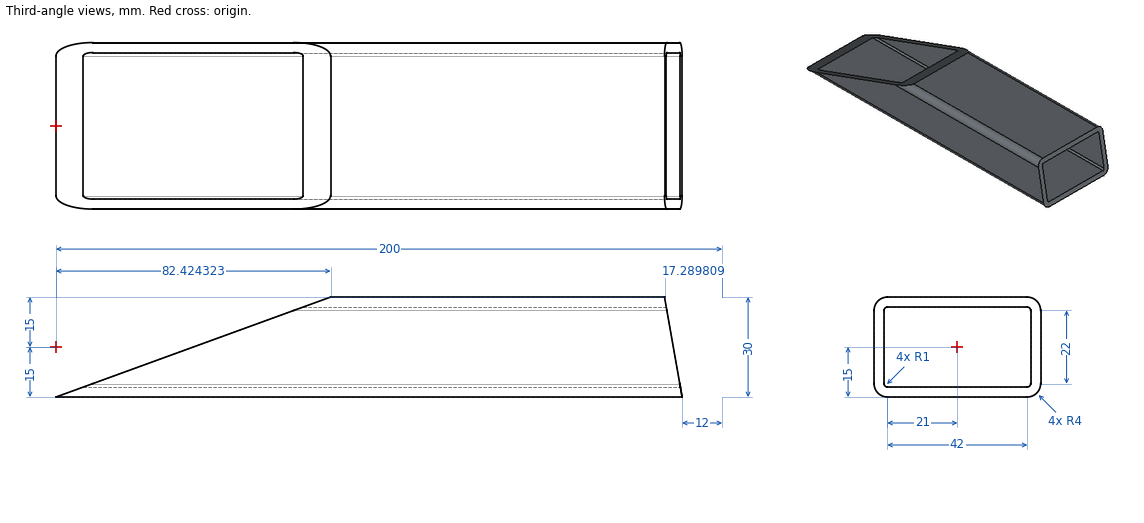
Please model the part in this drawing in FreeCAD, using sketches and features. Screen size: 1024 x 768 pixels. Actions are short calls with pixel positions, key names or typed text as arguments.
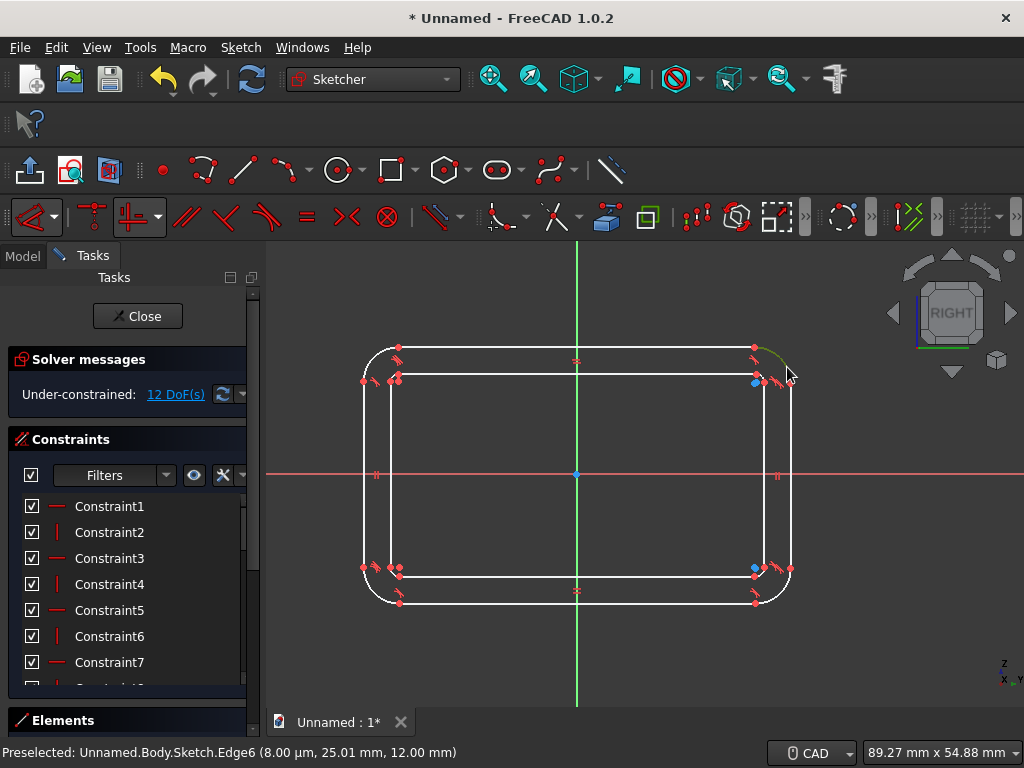
scroll(762, 377, up, 4)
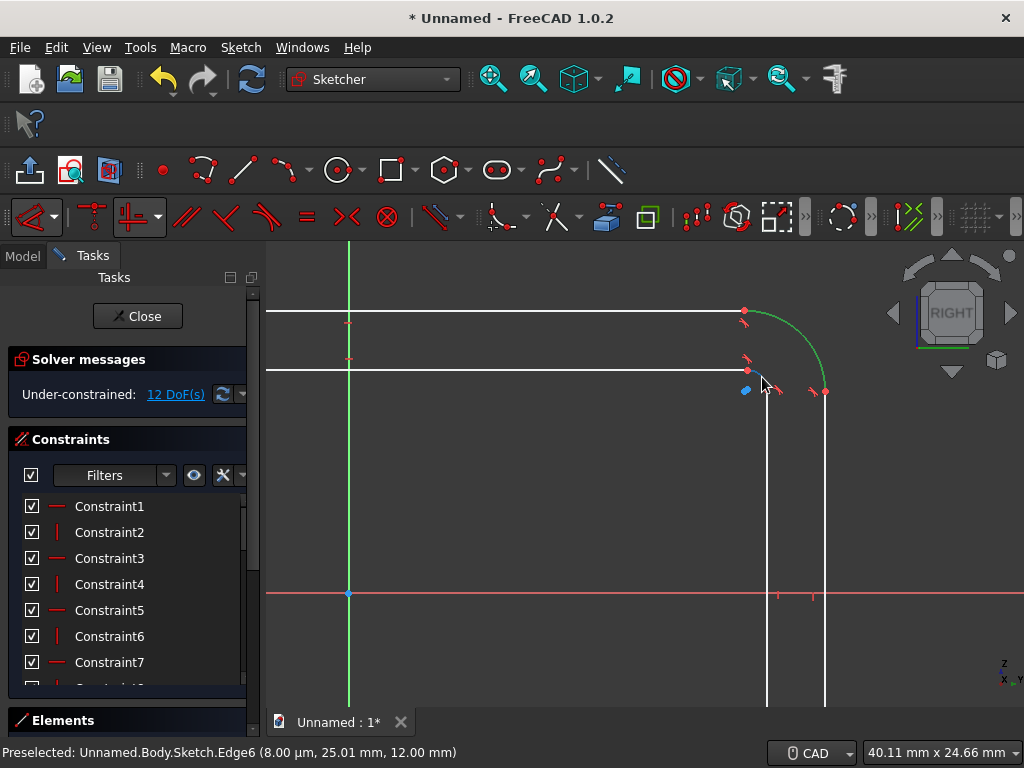
click(761, 376)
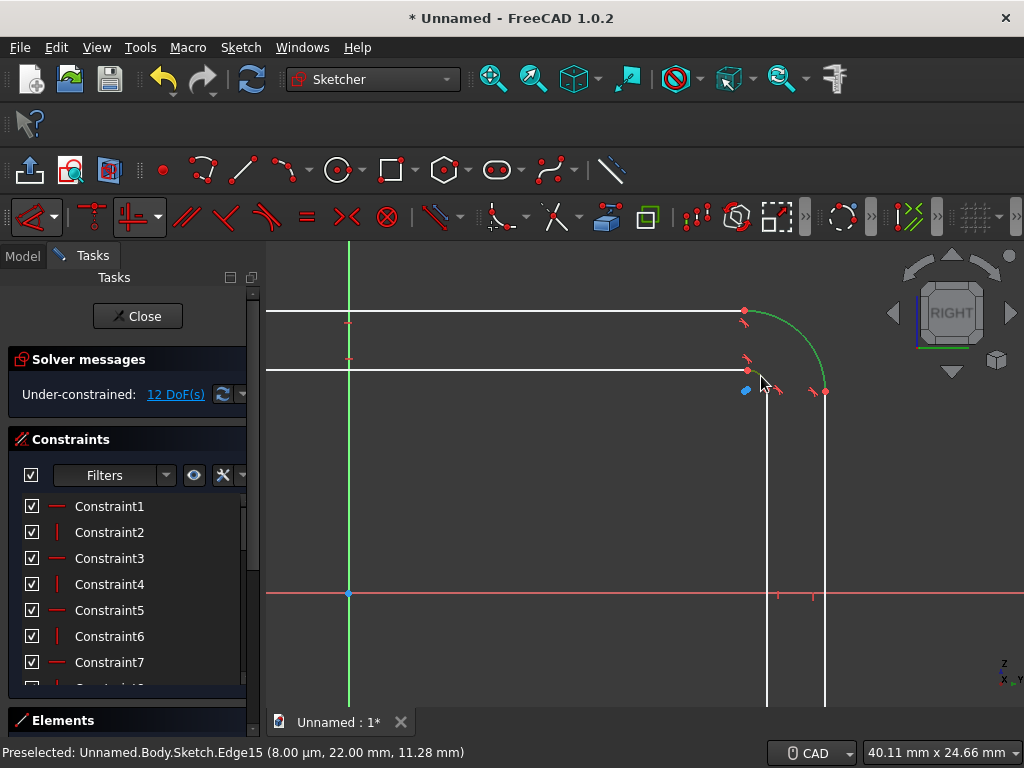
click(92, 218)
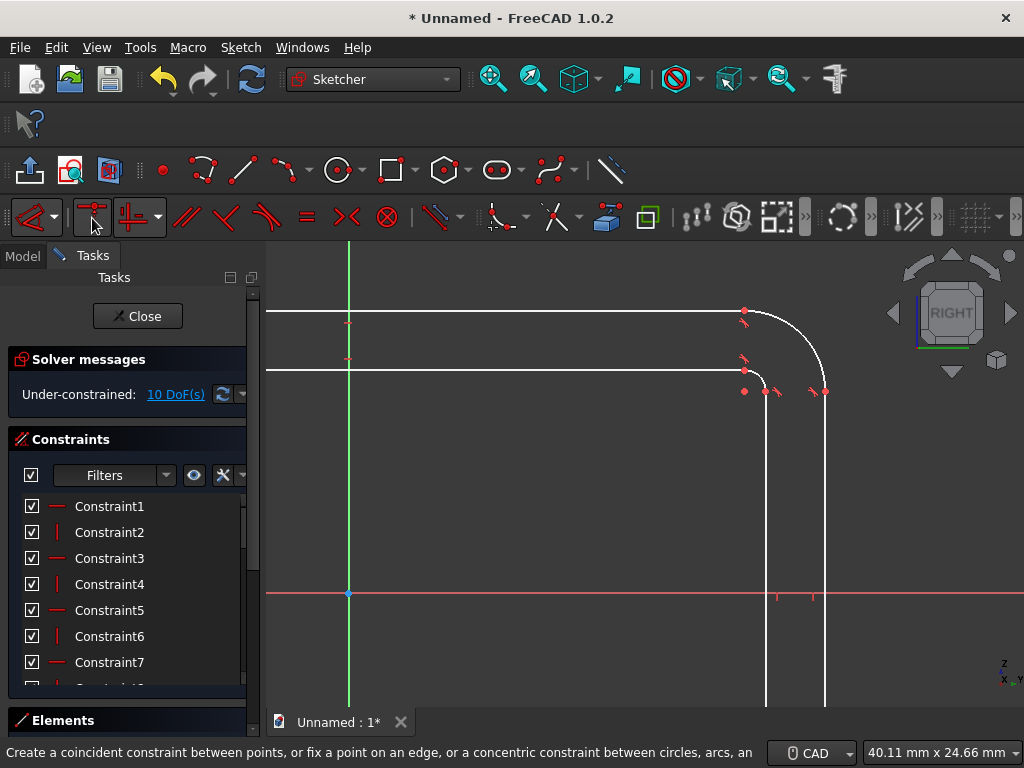
scroll(762, 377, down, 4)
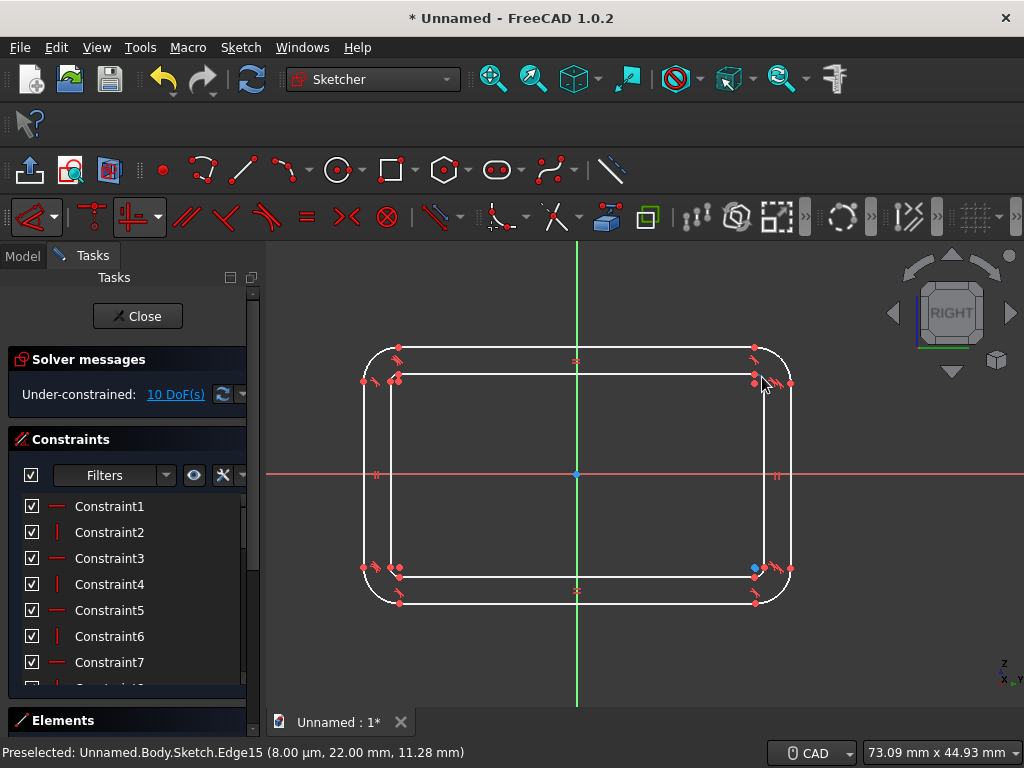
click(771, 600)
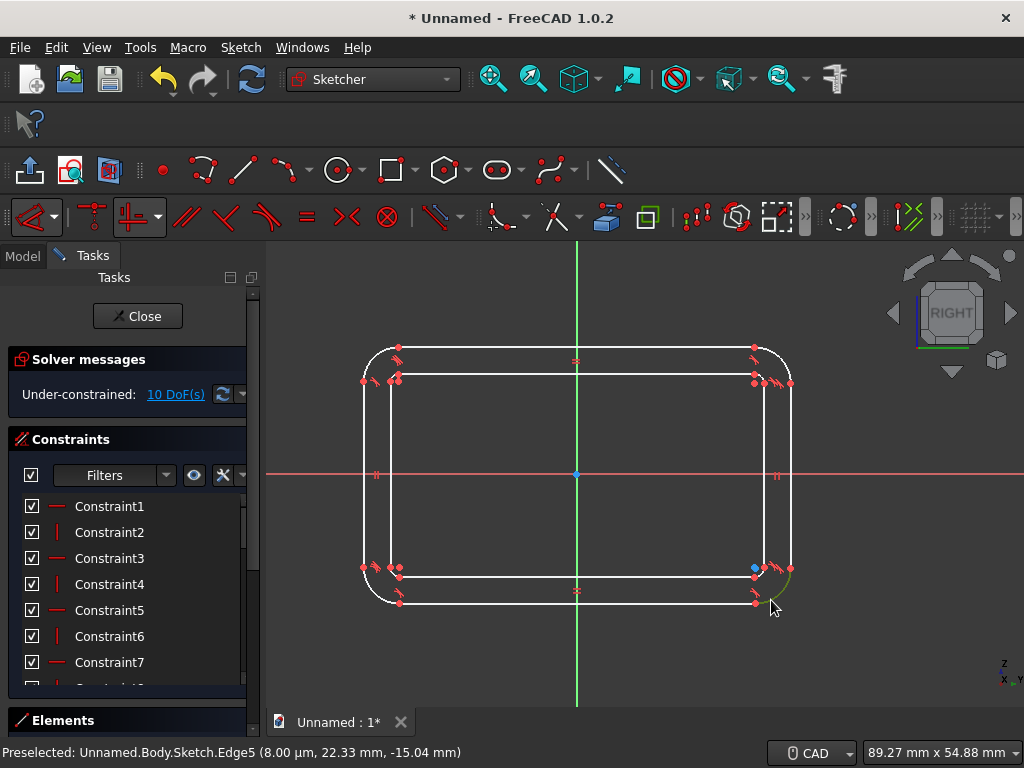
click(787, 367)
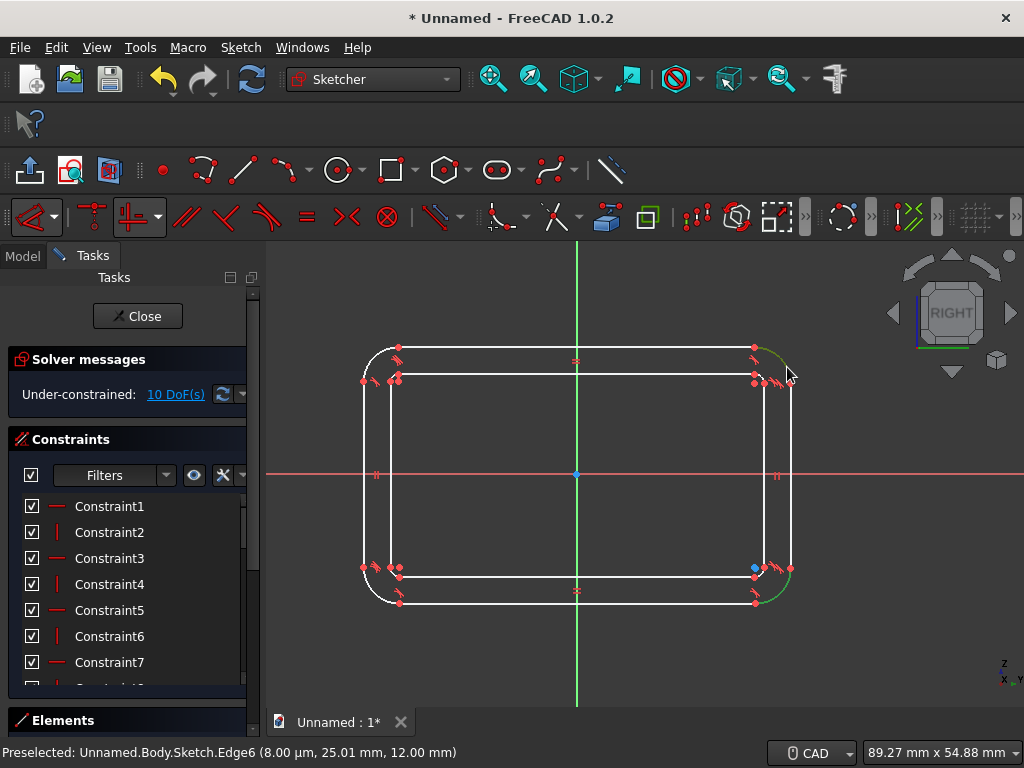
click(383, 351)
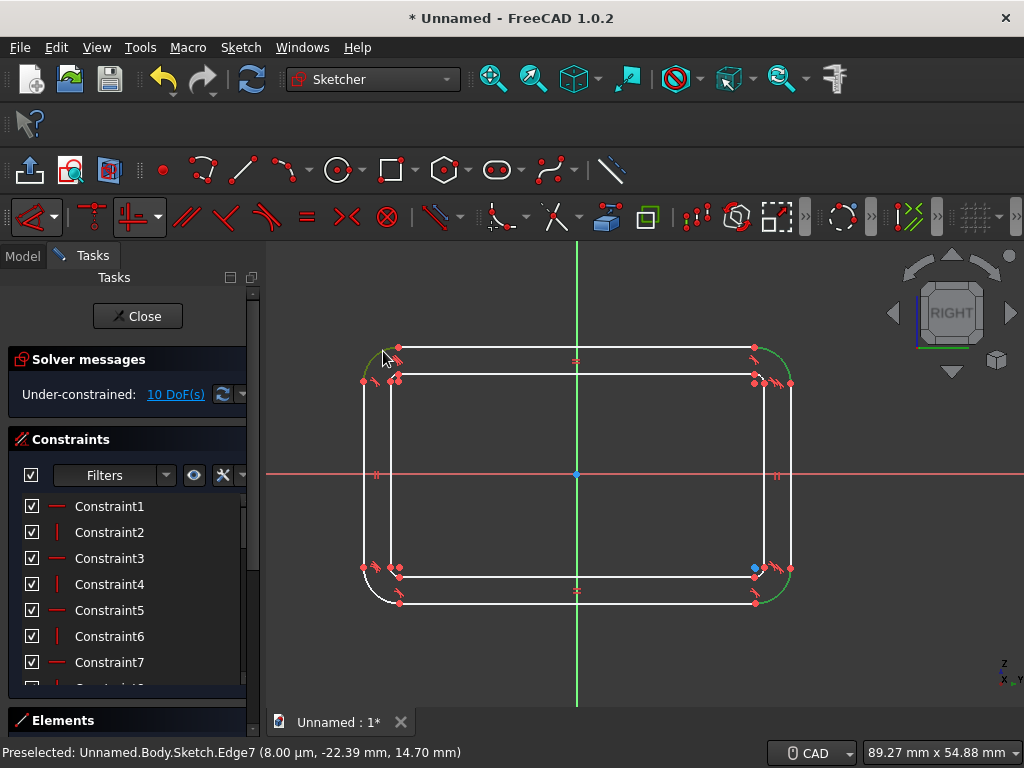
click(368, 584)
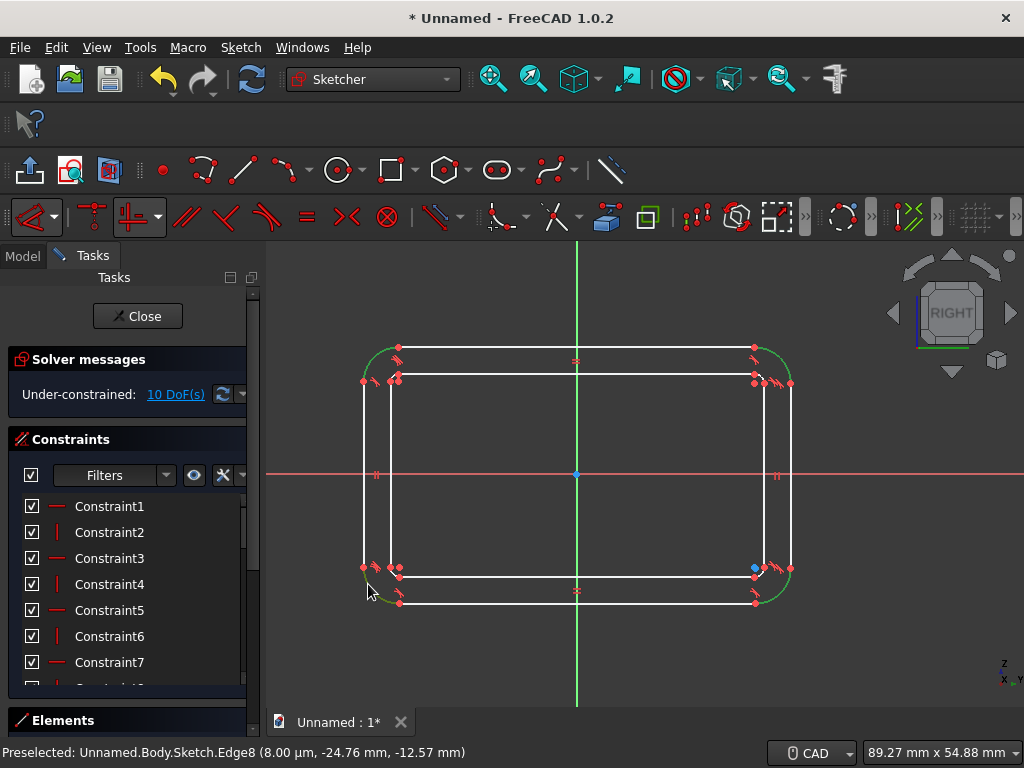
click(308, 218)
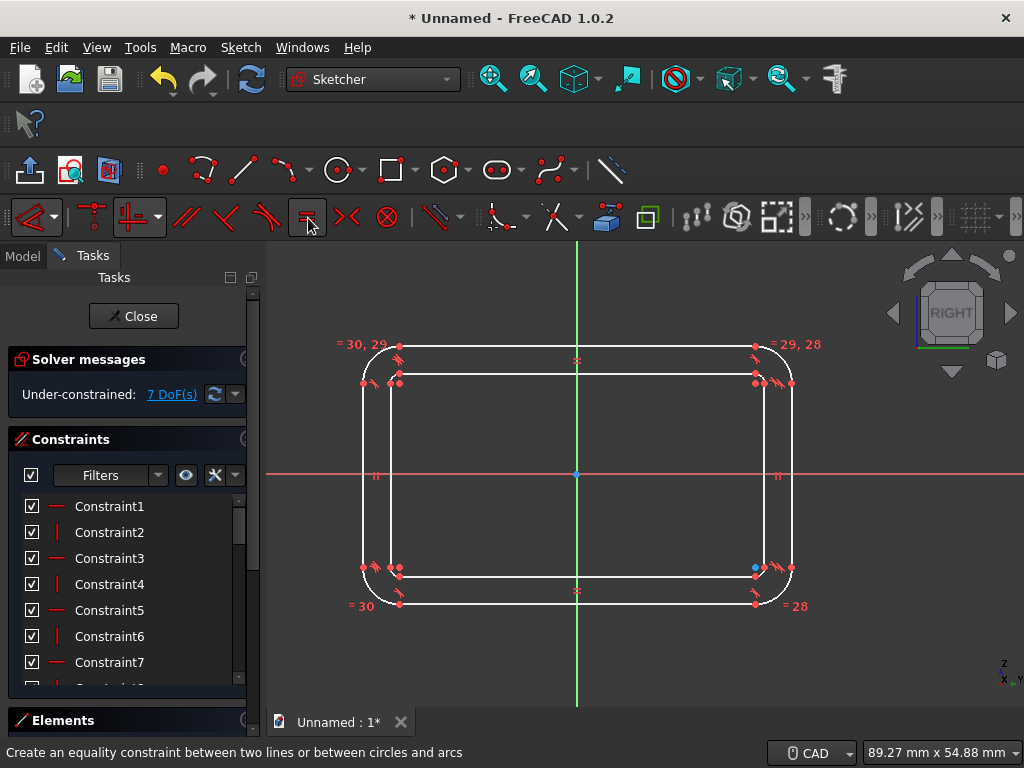
scroll(393, 574, up, 4)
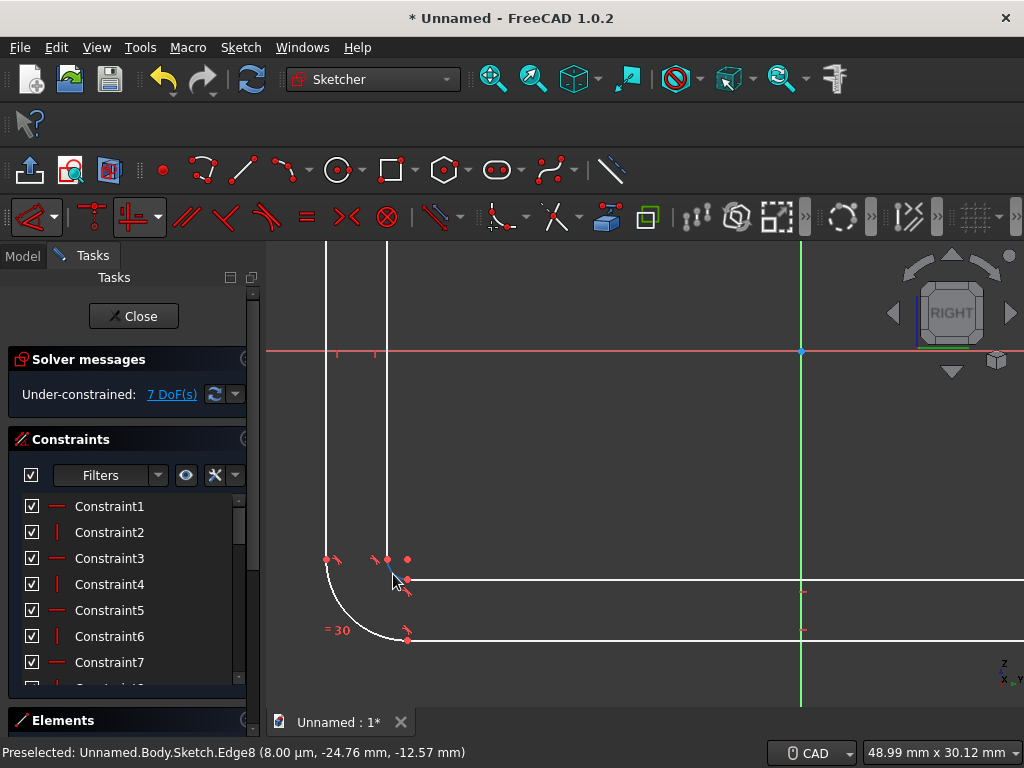
click(393, 574)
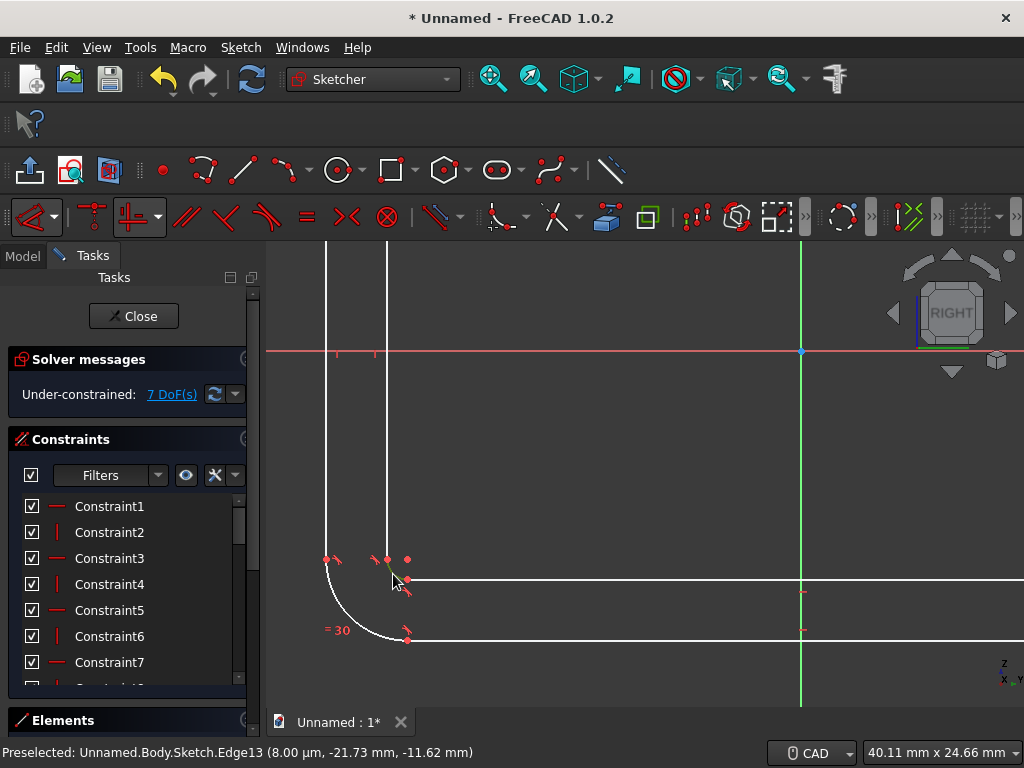
scroll(393, 574, down, 4)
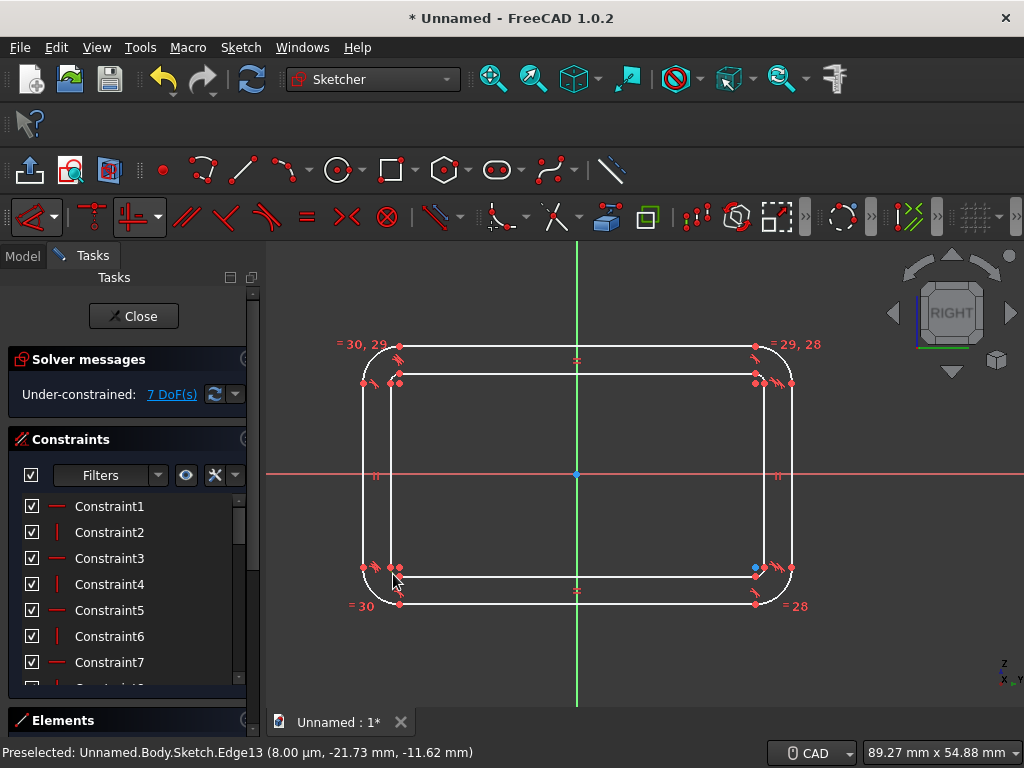
scroll(759, 576, up, 6)